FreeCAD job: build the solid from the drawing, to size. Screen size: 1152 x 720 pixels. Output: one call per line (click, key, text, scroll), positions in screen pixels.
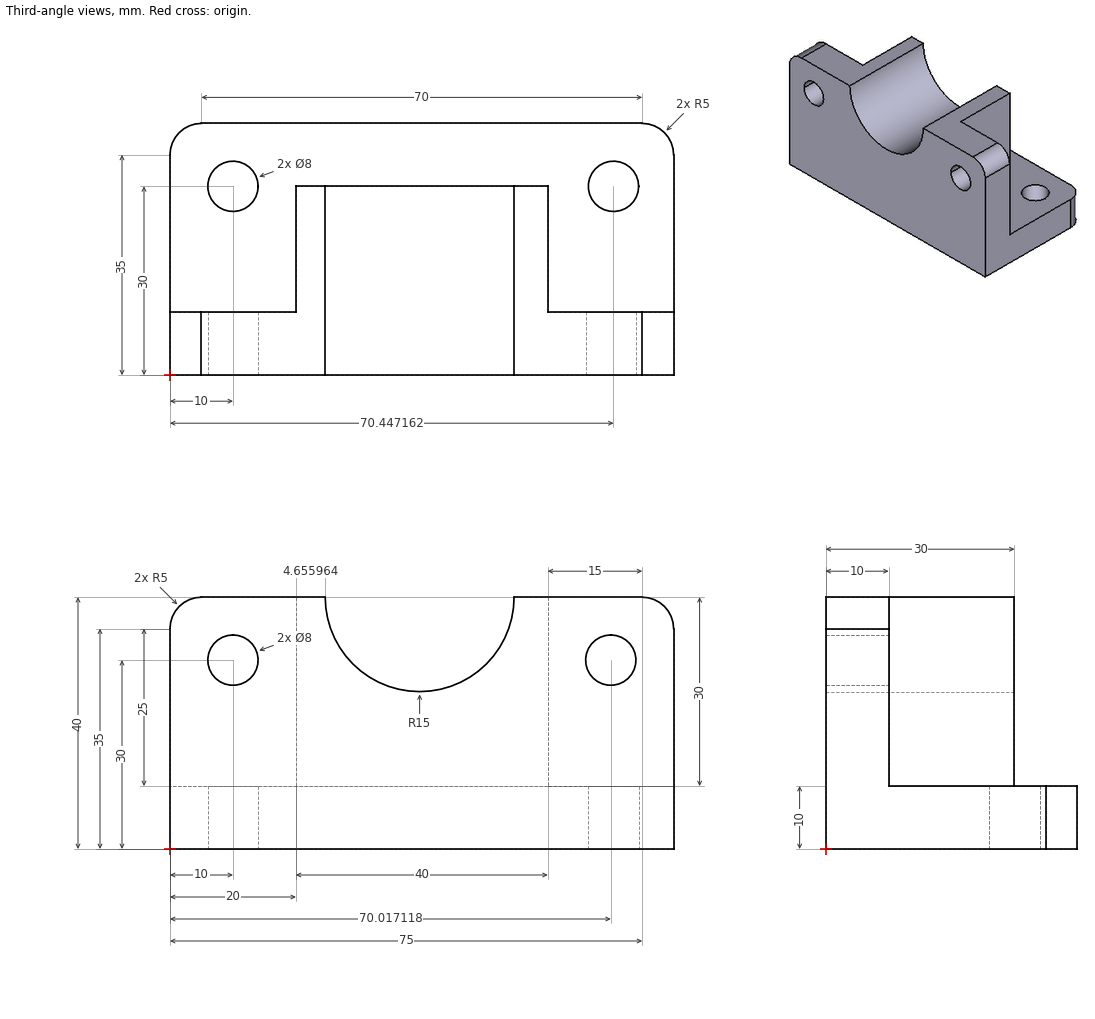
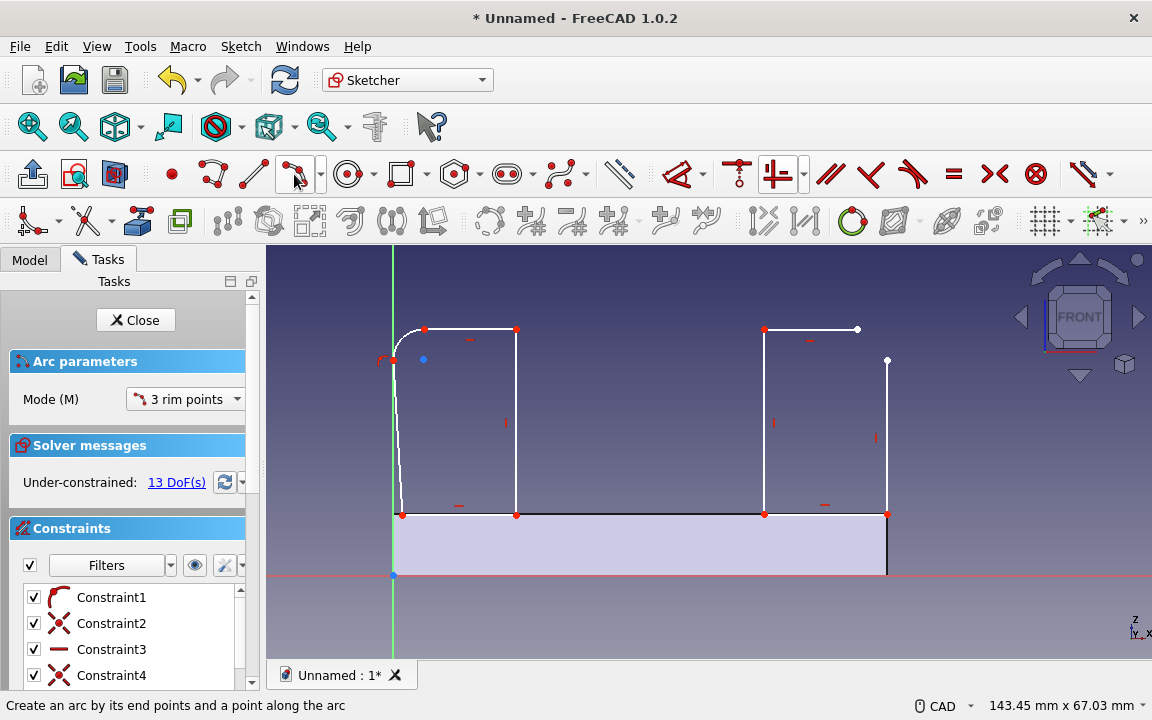
click(887, 361)
click(857, 330)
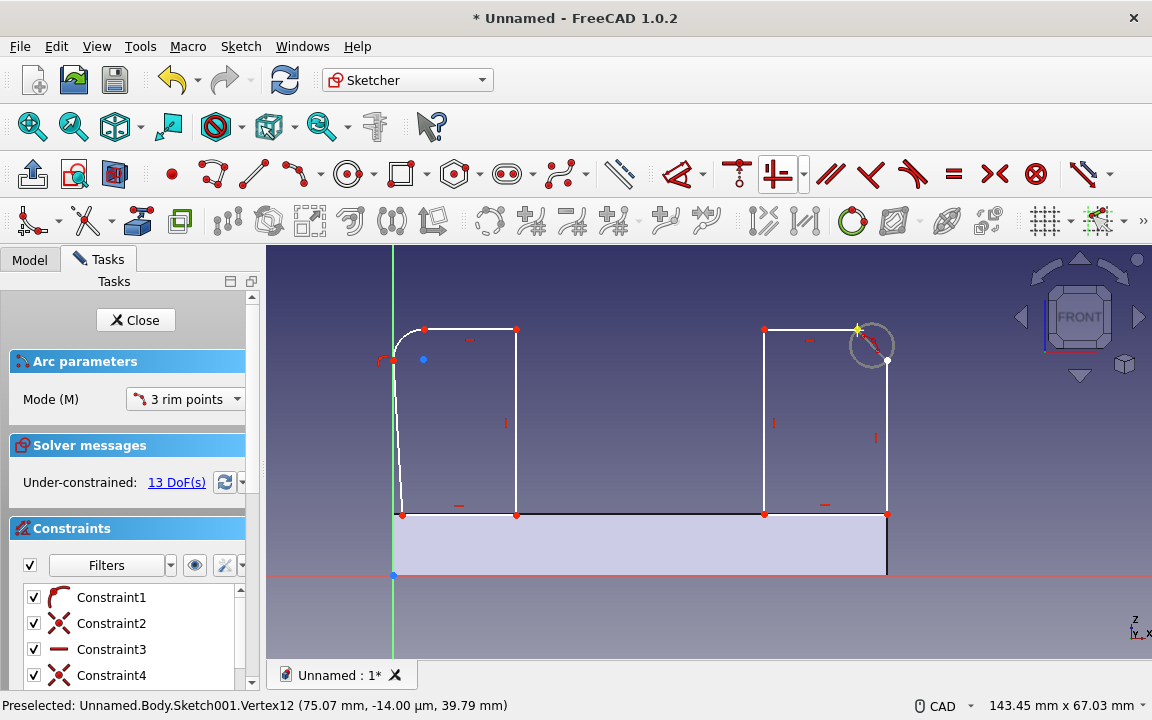
scroll(878, 338, up, 3)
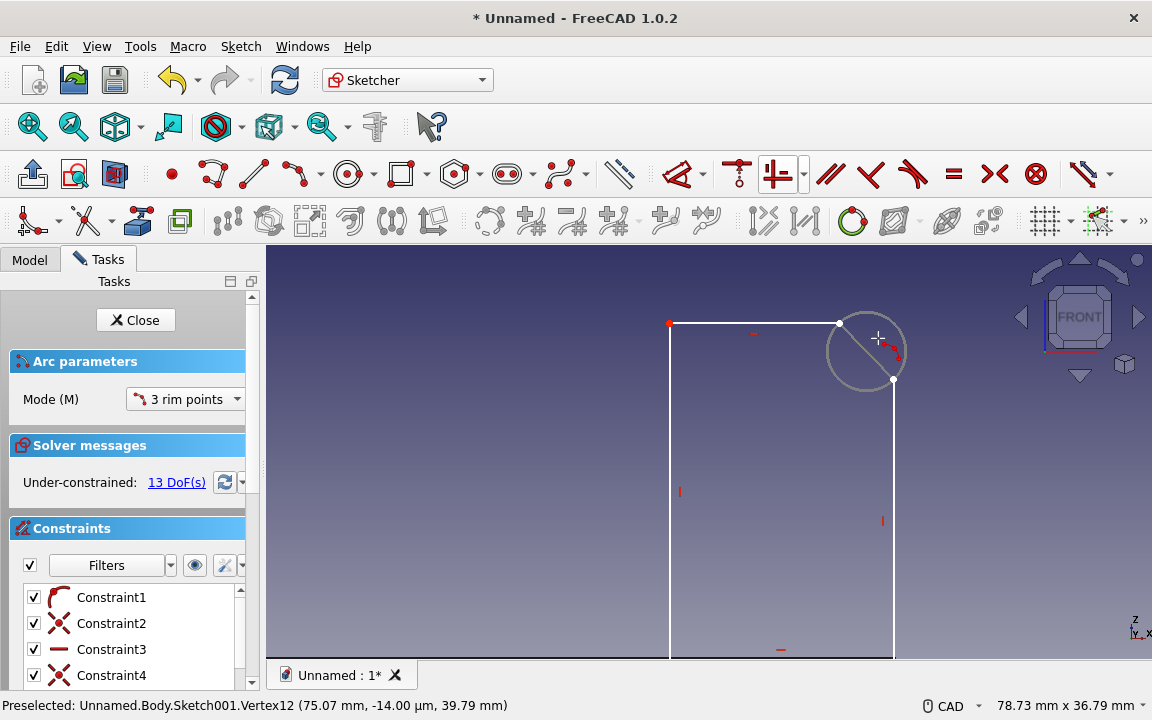
click(878, 337)
key(Escape)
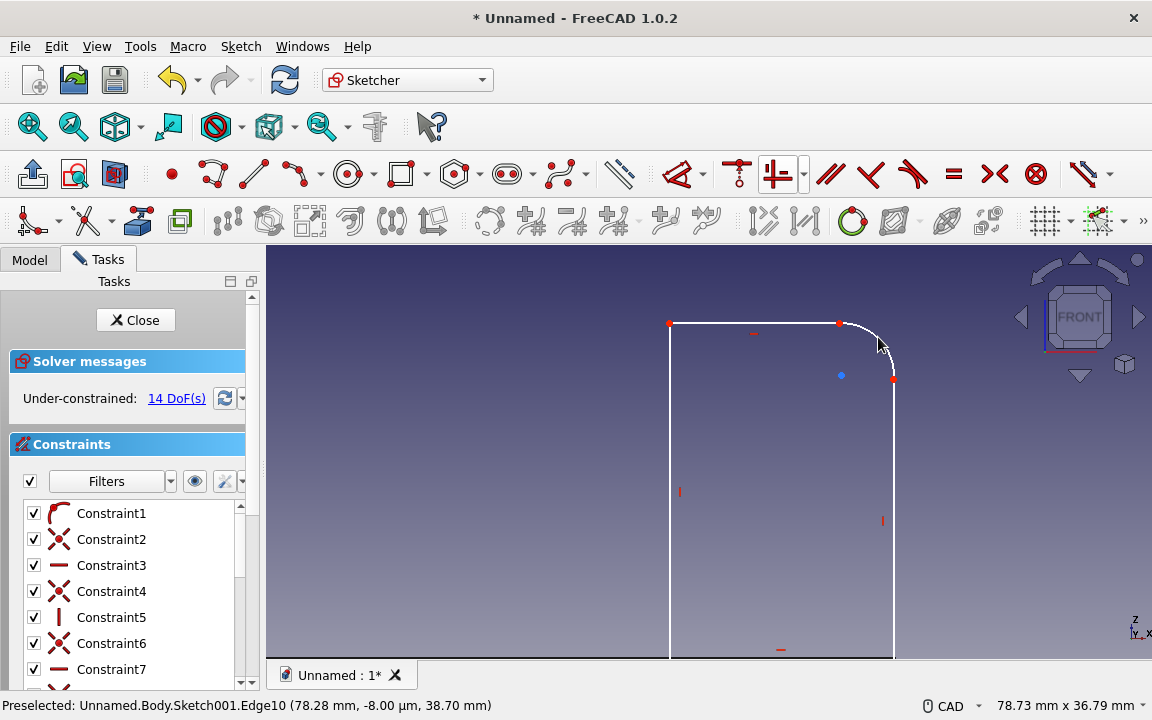
scroll(879, 338, down, 3)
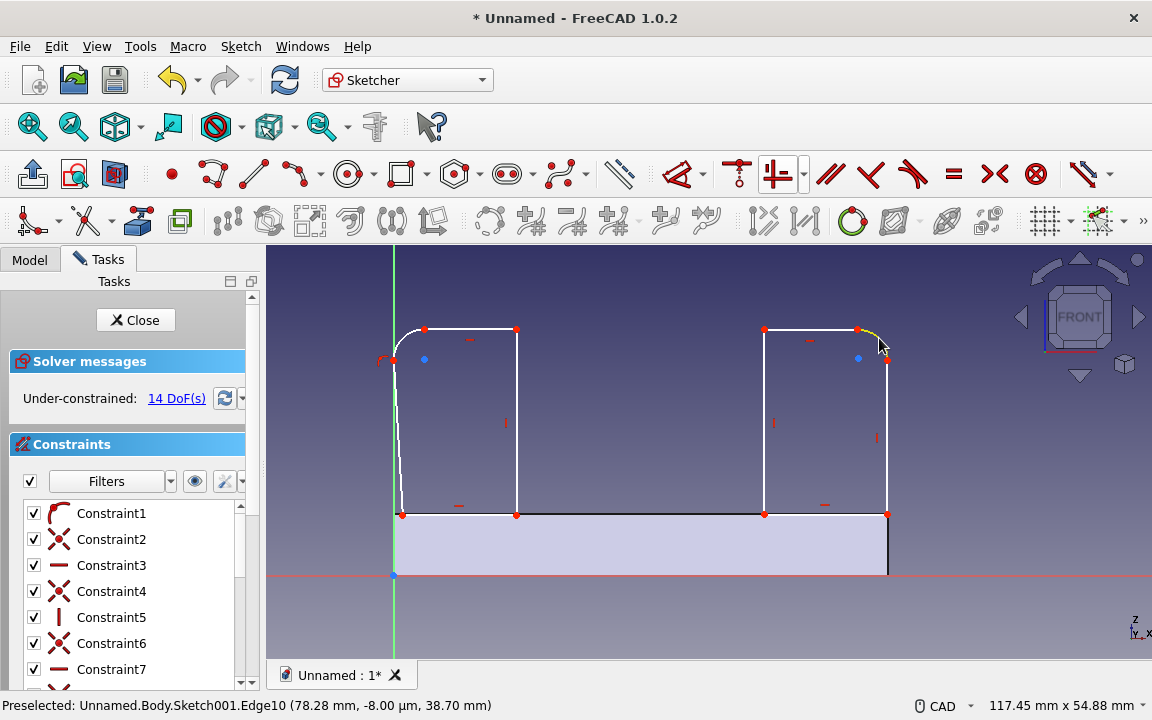
scroll(400, 469, up, 4)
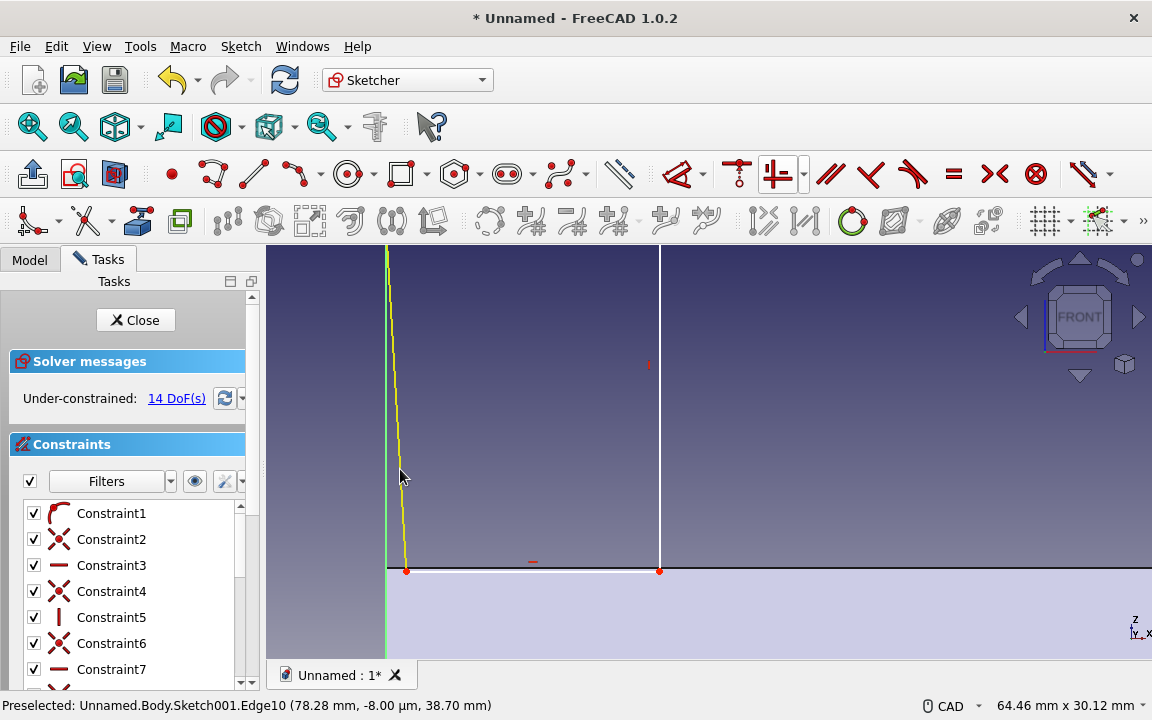
click(400, 468)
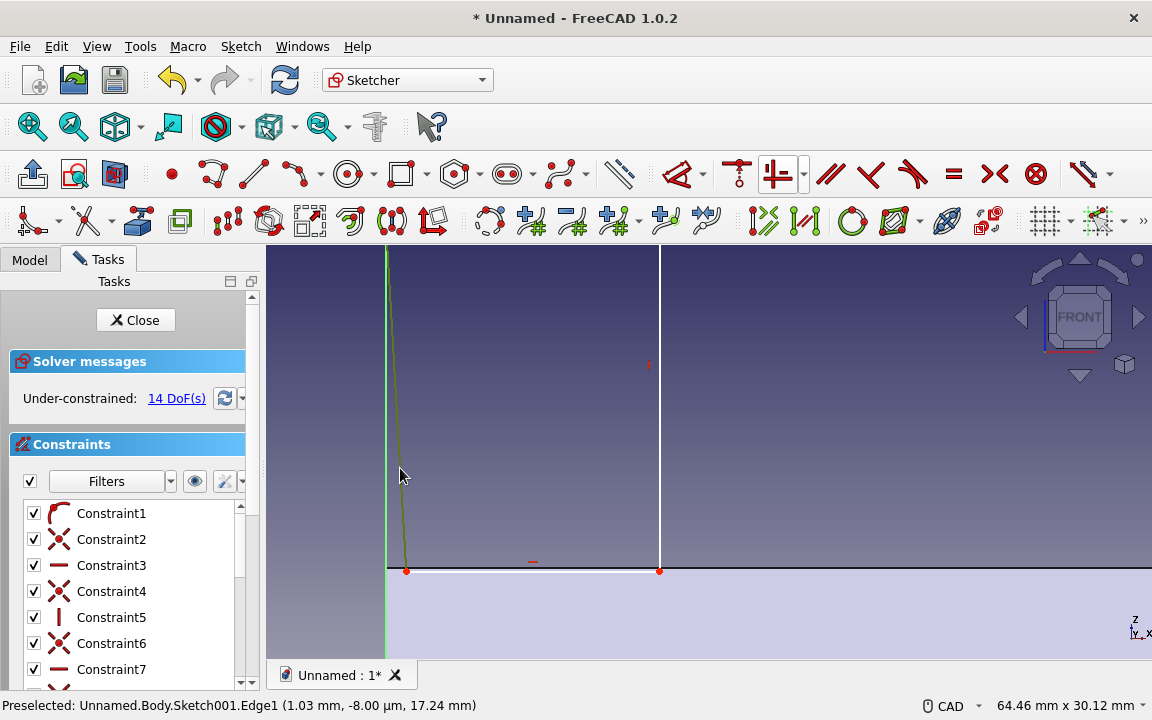
scroll(399, 469, down, 4)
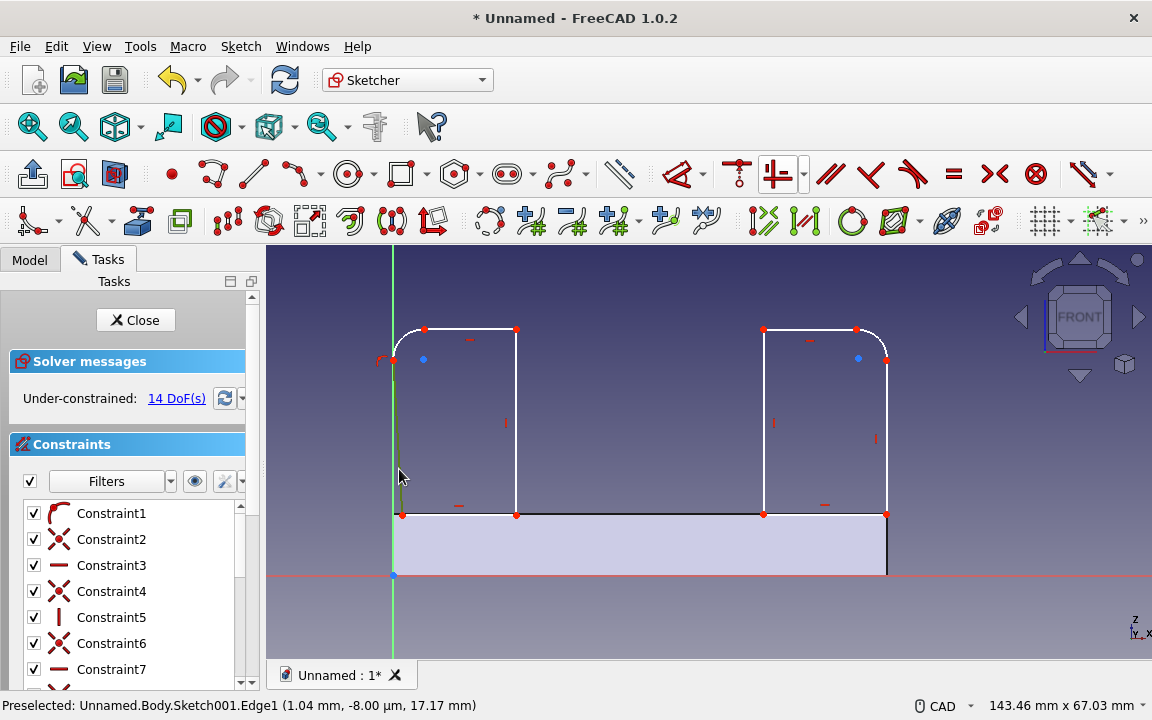
click(410, 333)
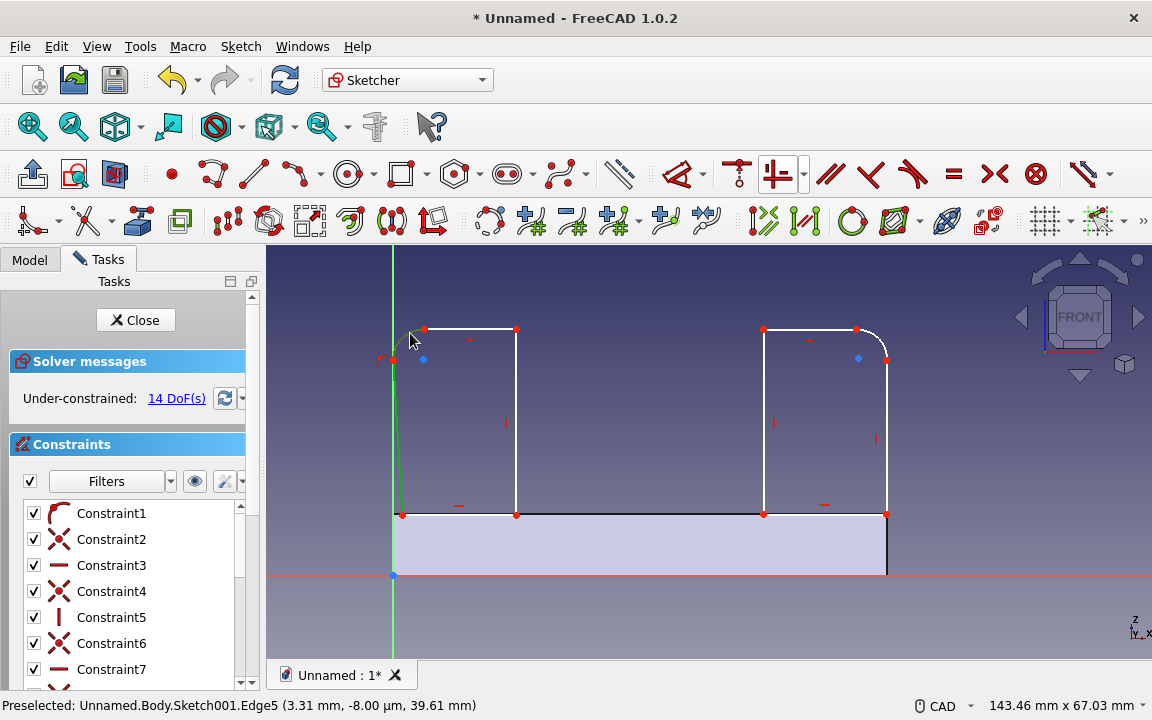
click(913, 174)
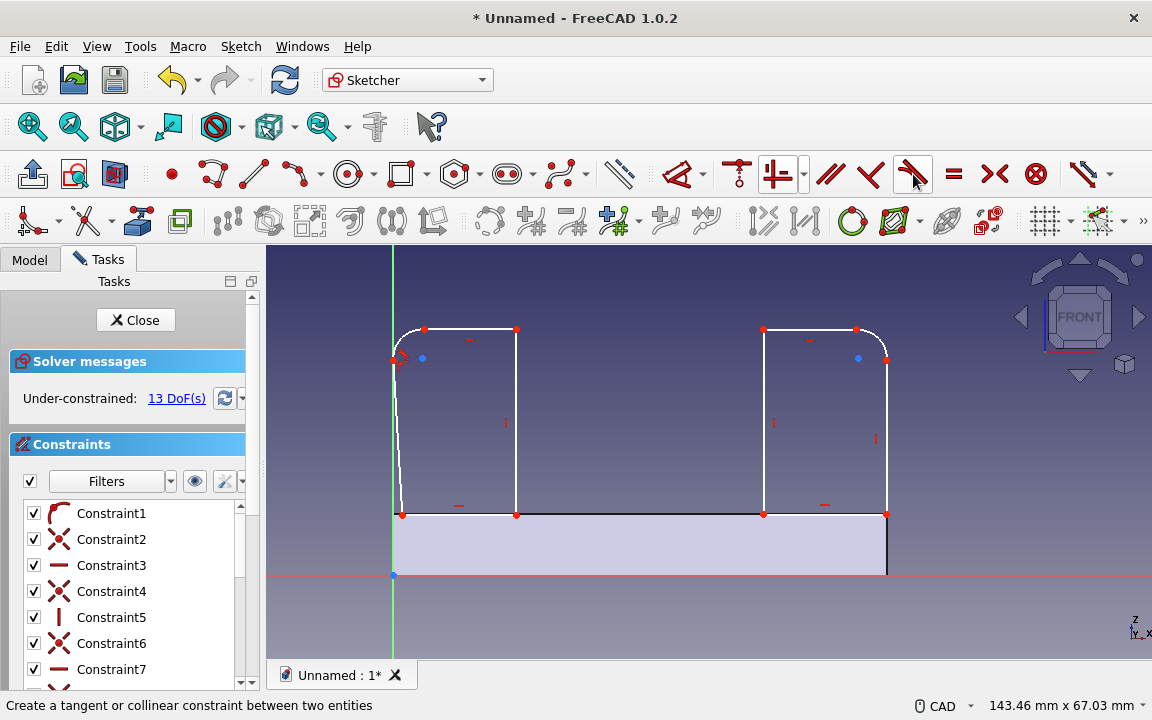
click(489, 329)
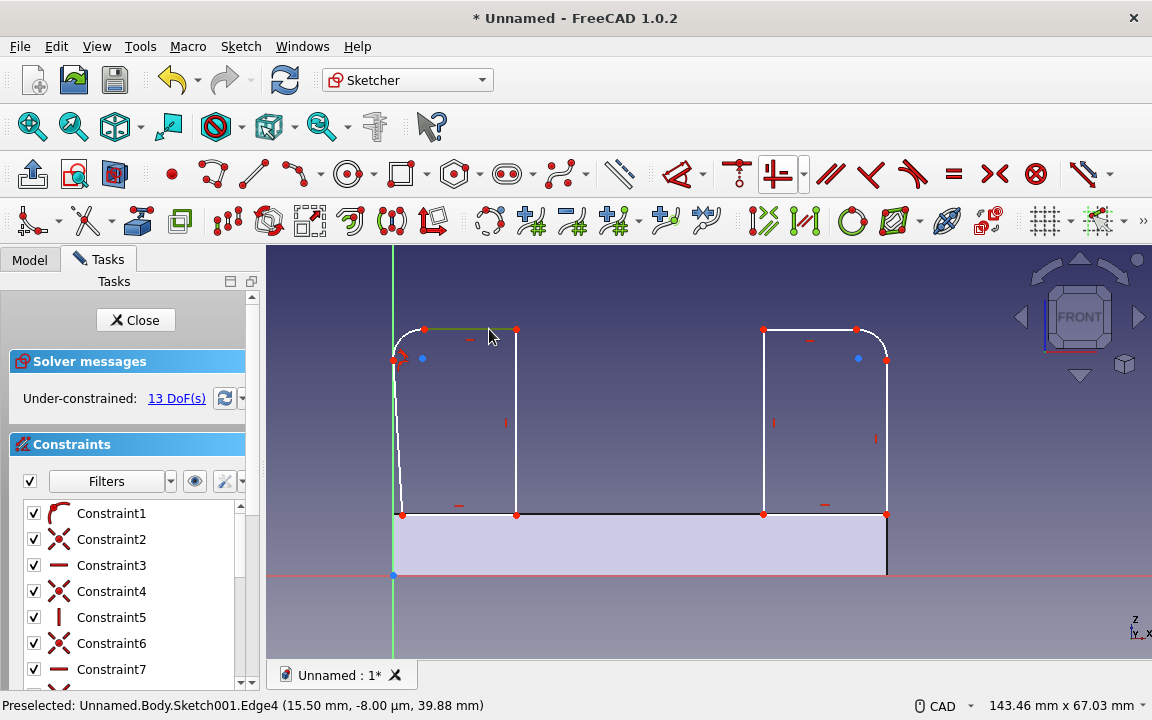
click(410, 332)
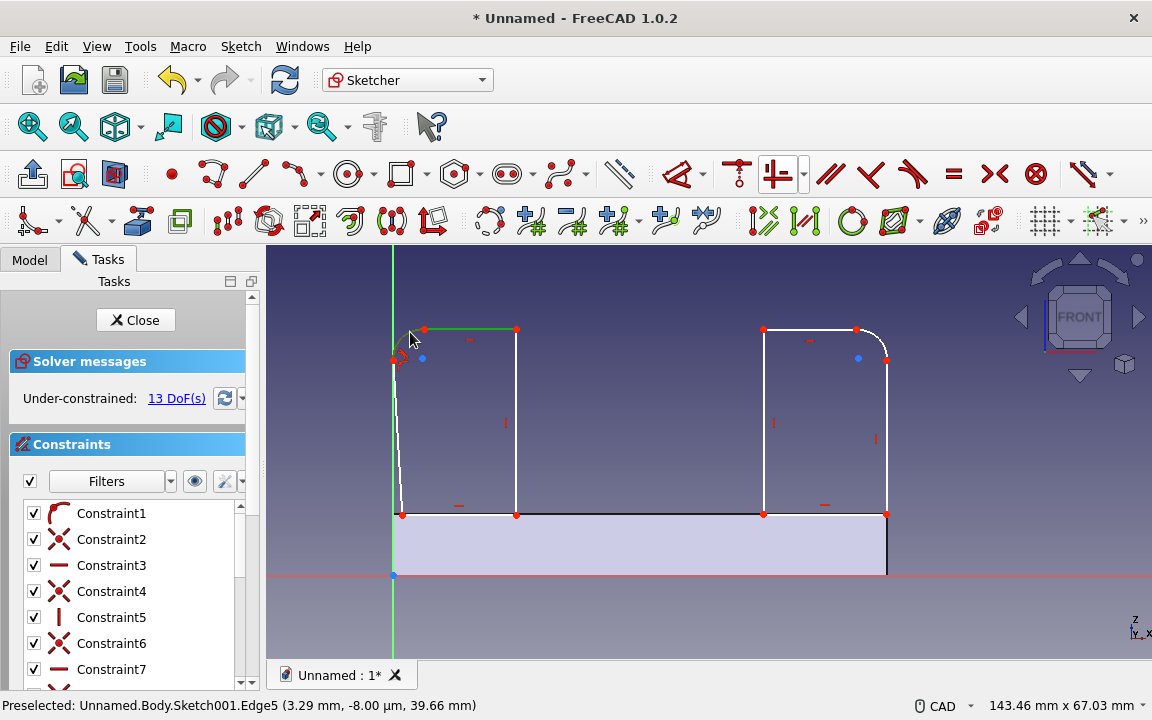
key(t)